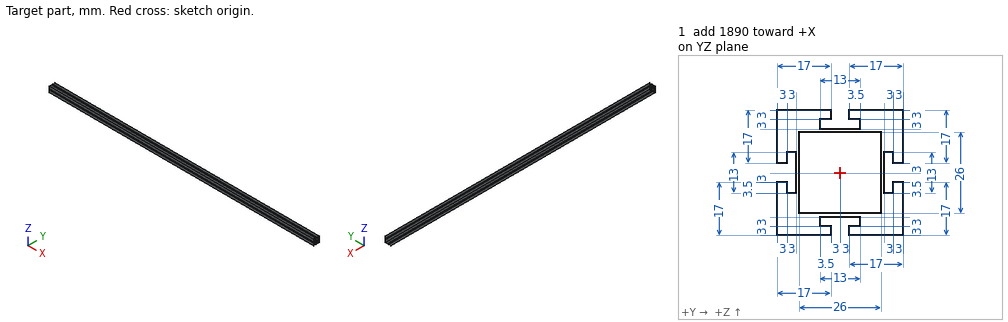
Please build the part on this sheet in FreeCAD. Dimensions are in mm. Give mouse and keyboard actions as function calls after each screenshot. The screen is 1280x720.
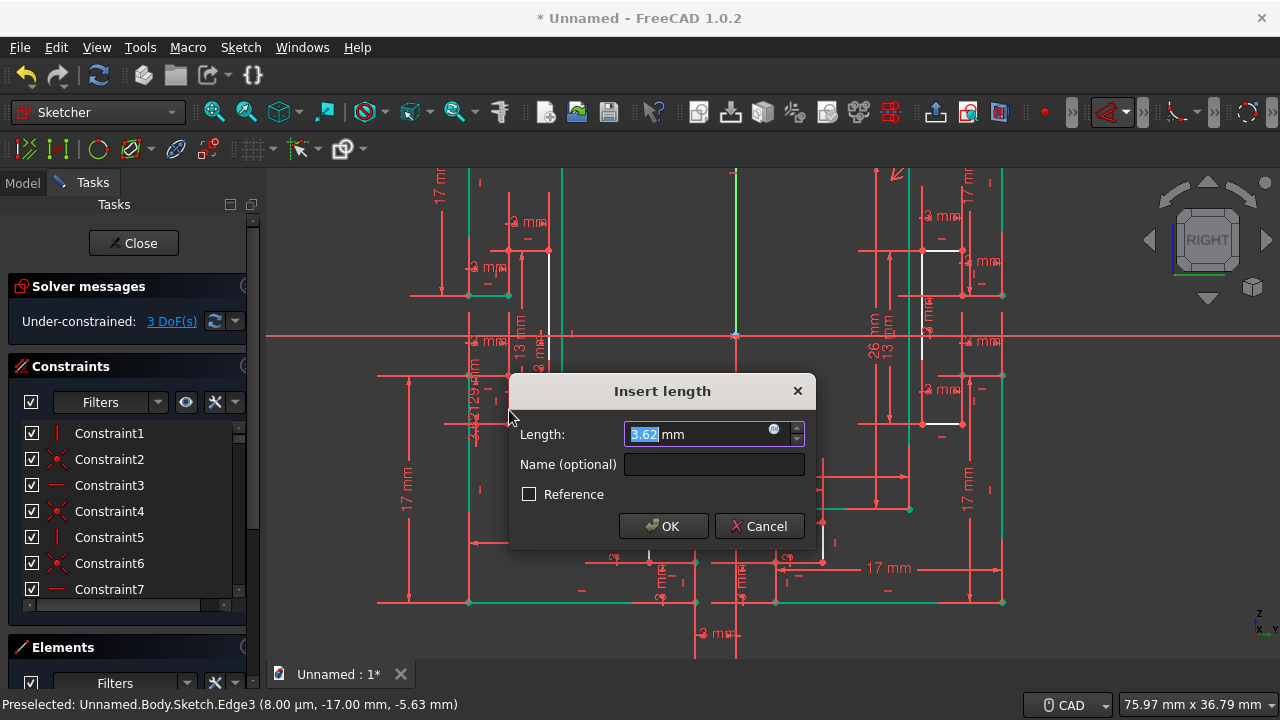
text(3.5)
key(Return)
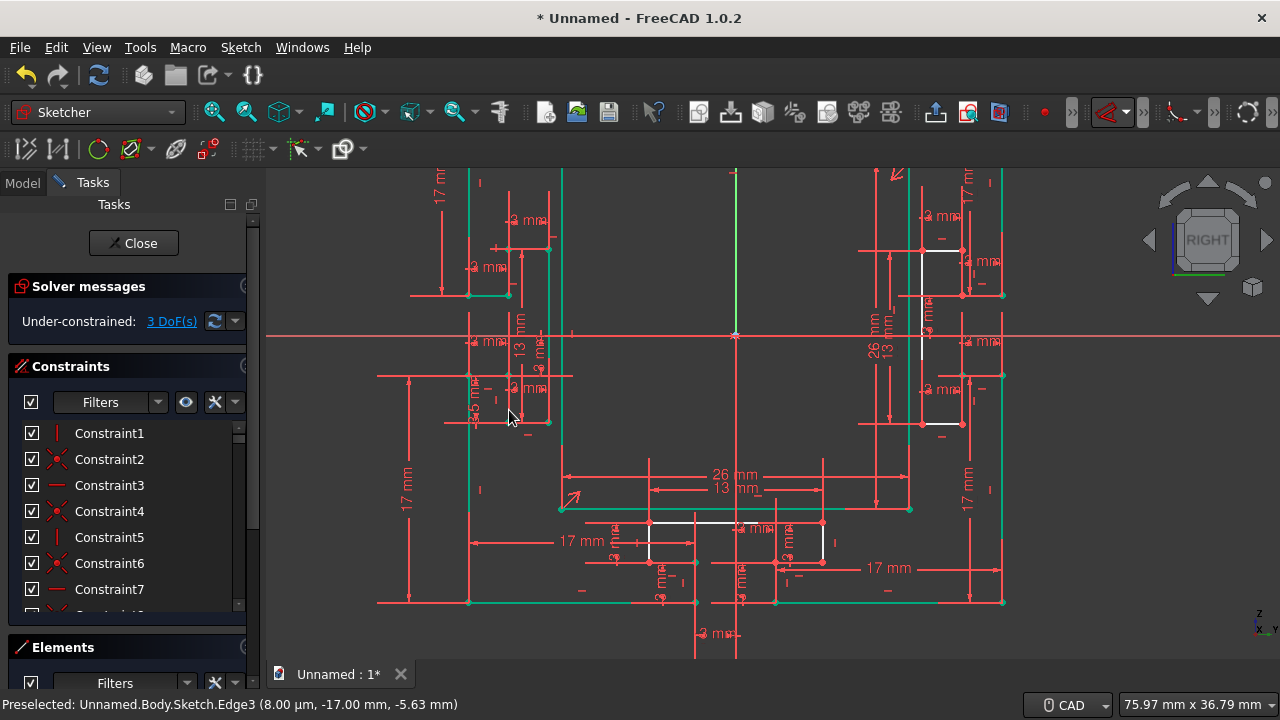
click(682, 563)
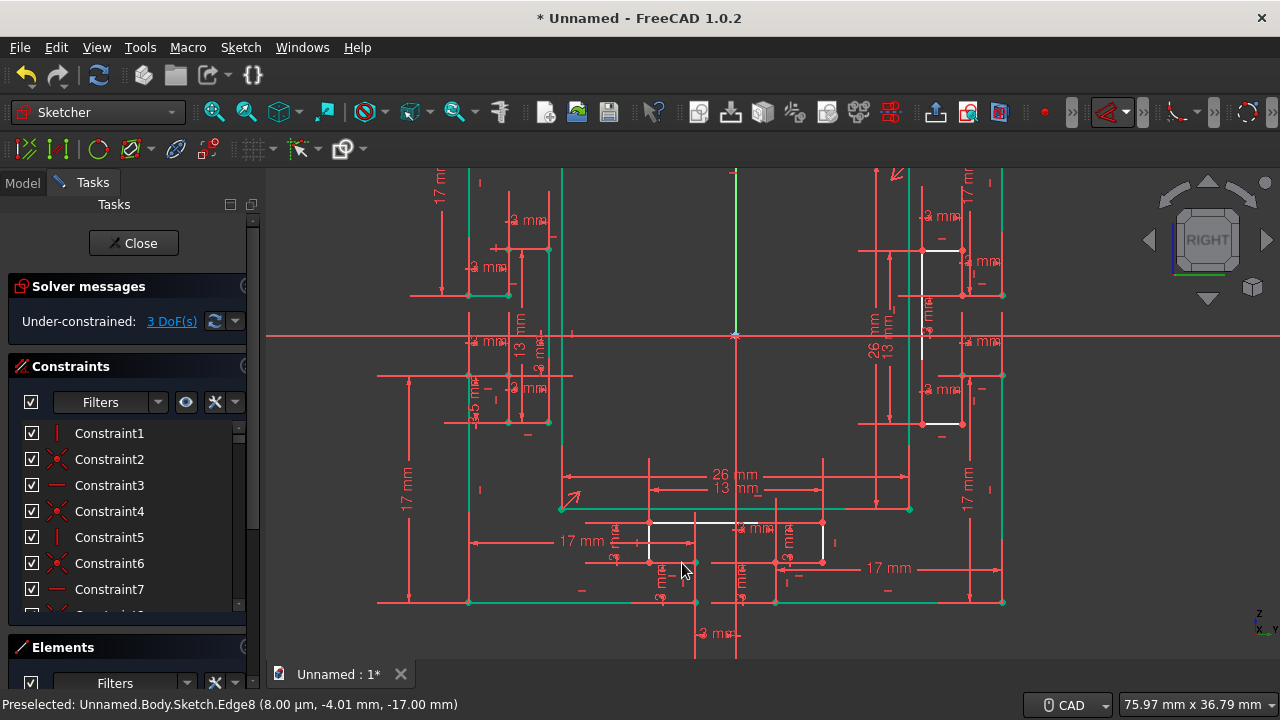
key(l)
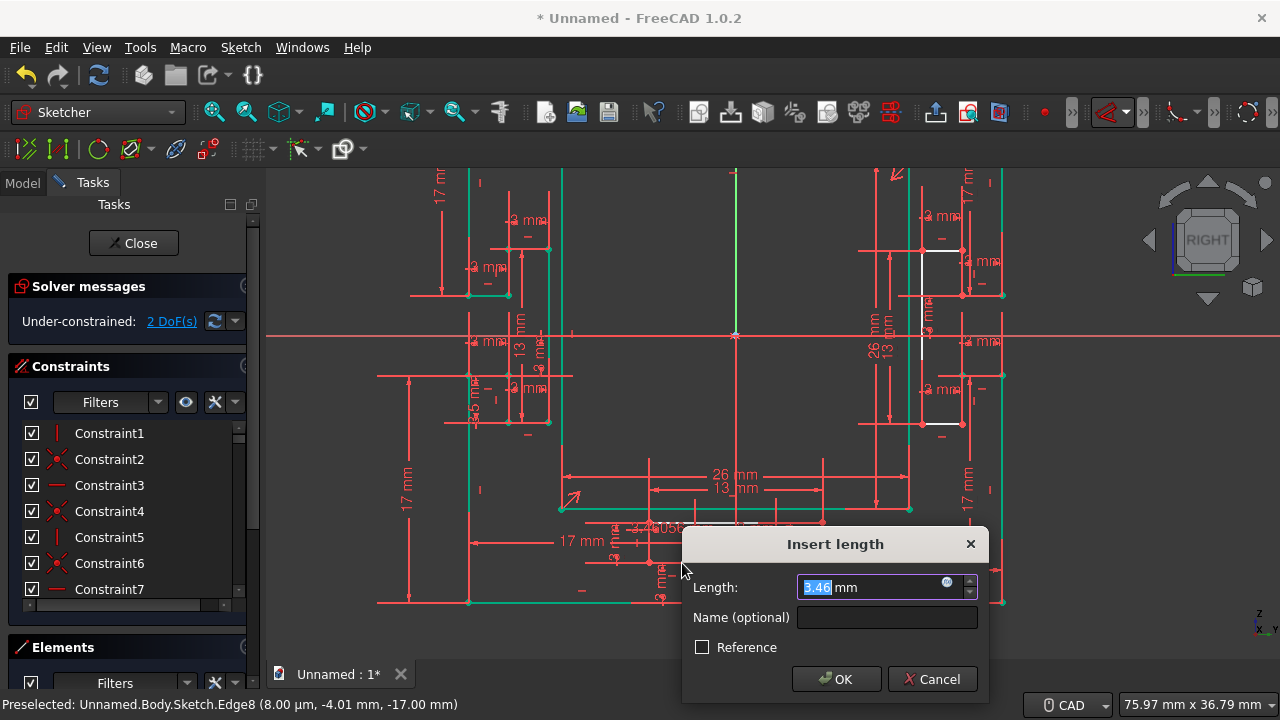
text(3.5)
key(Return)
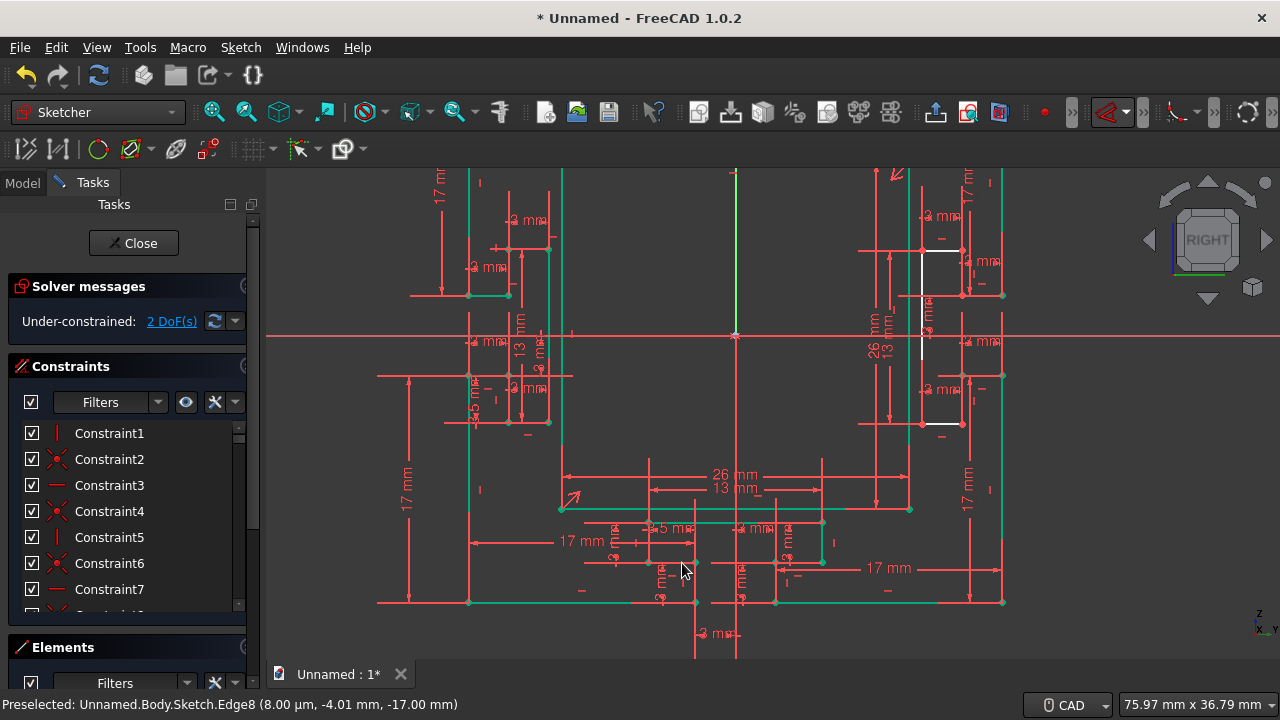
click(962, 390)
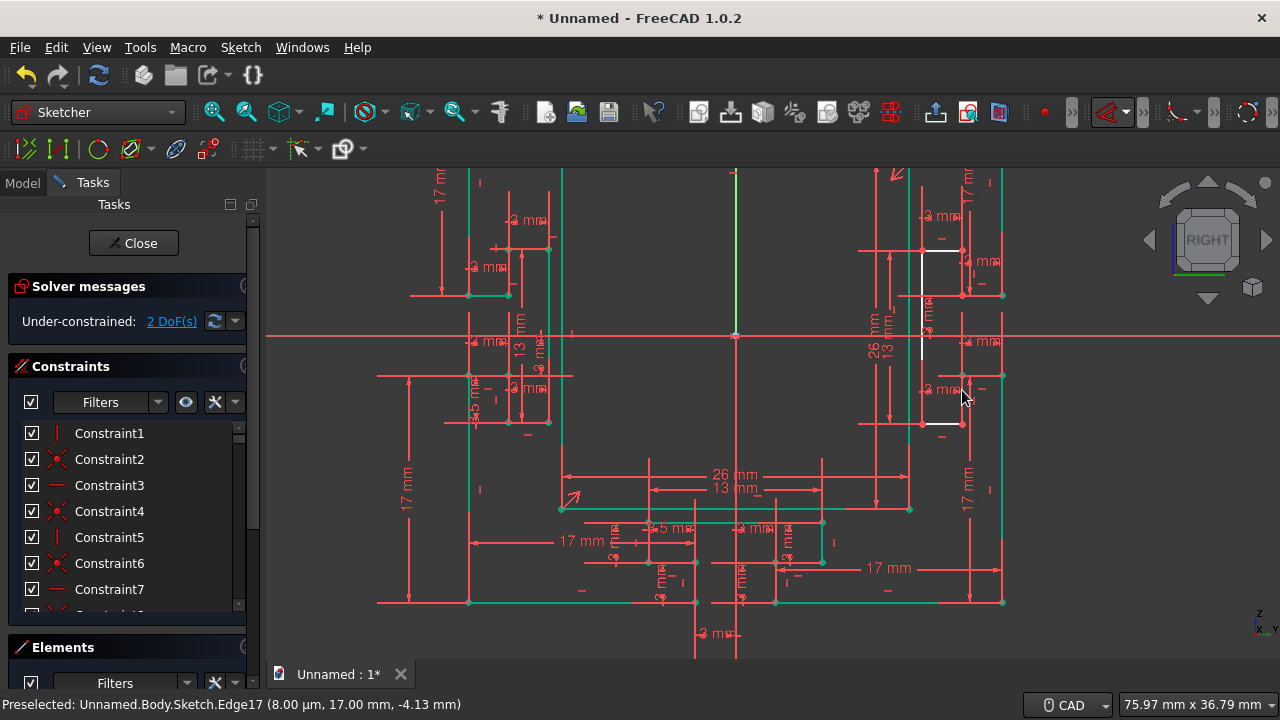
key(i)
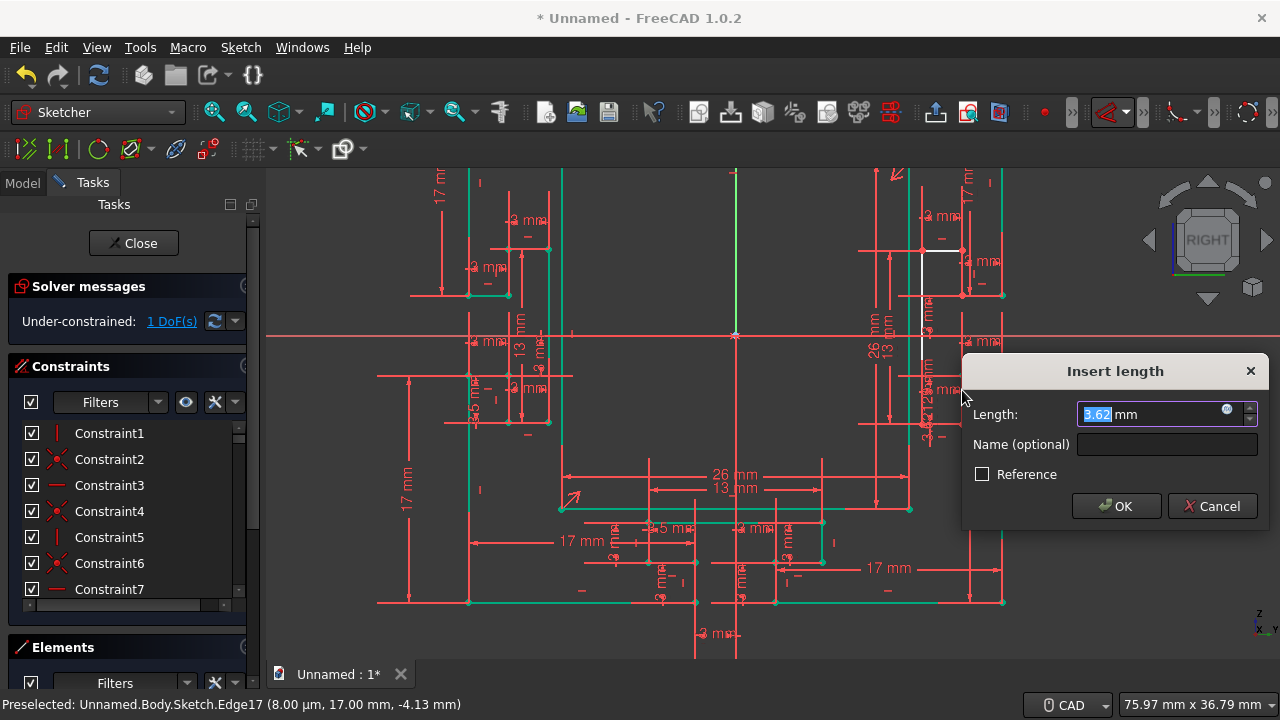
text(3.5)
key(Return)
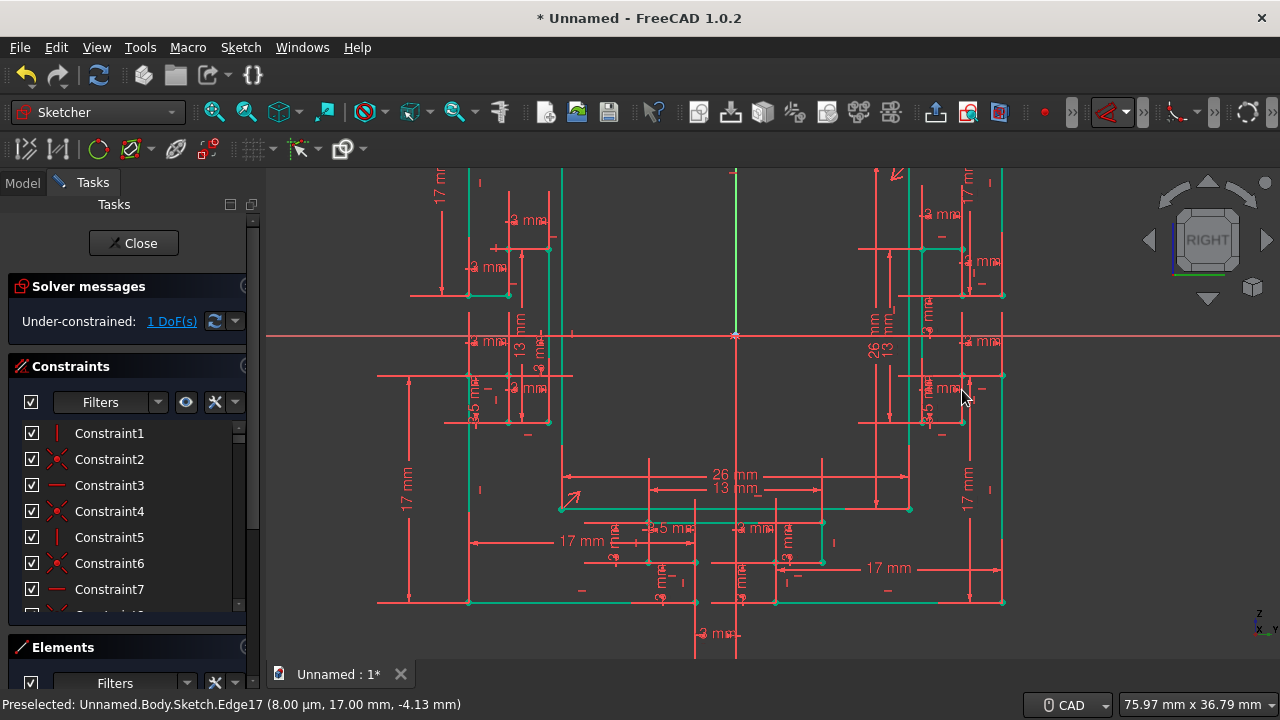
scroll(667, 508, down, 3)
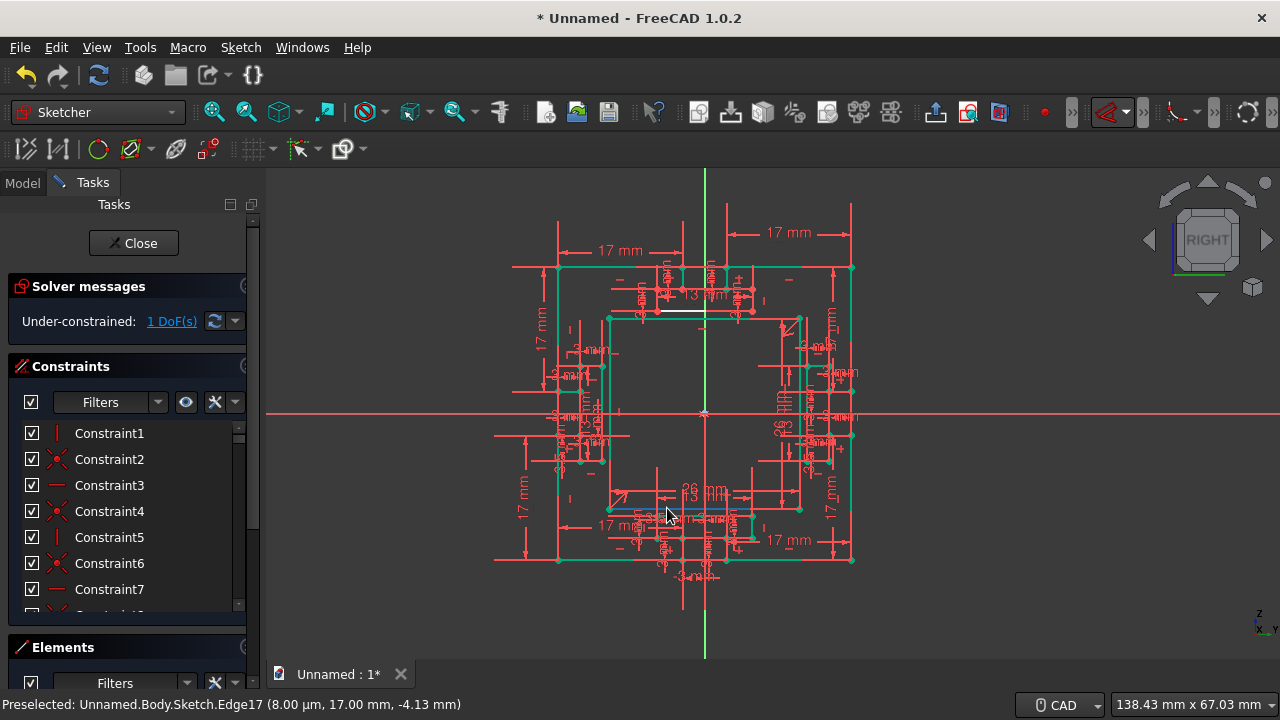
scroll(735, 289, up, 3)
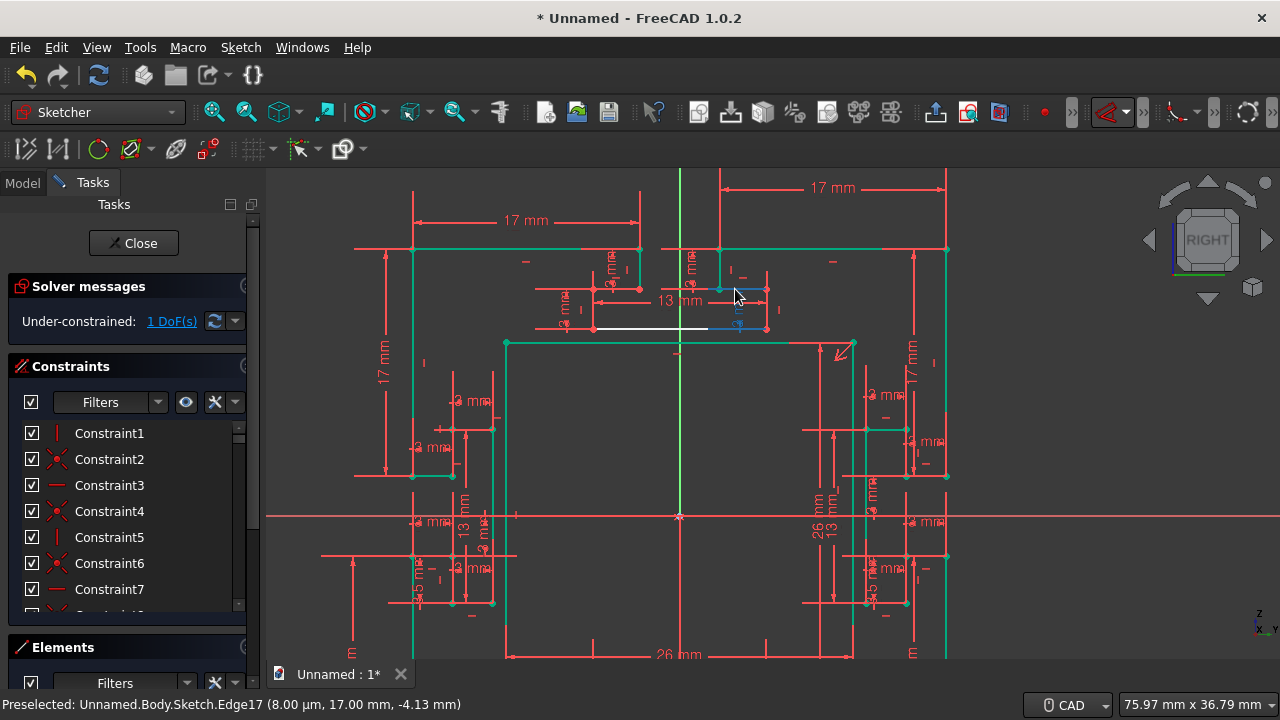
click(734, 289)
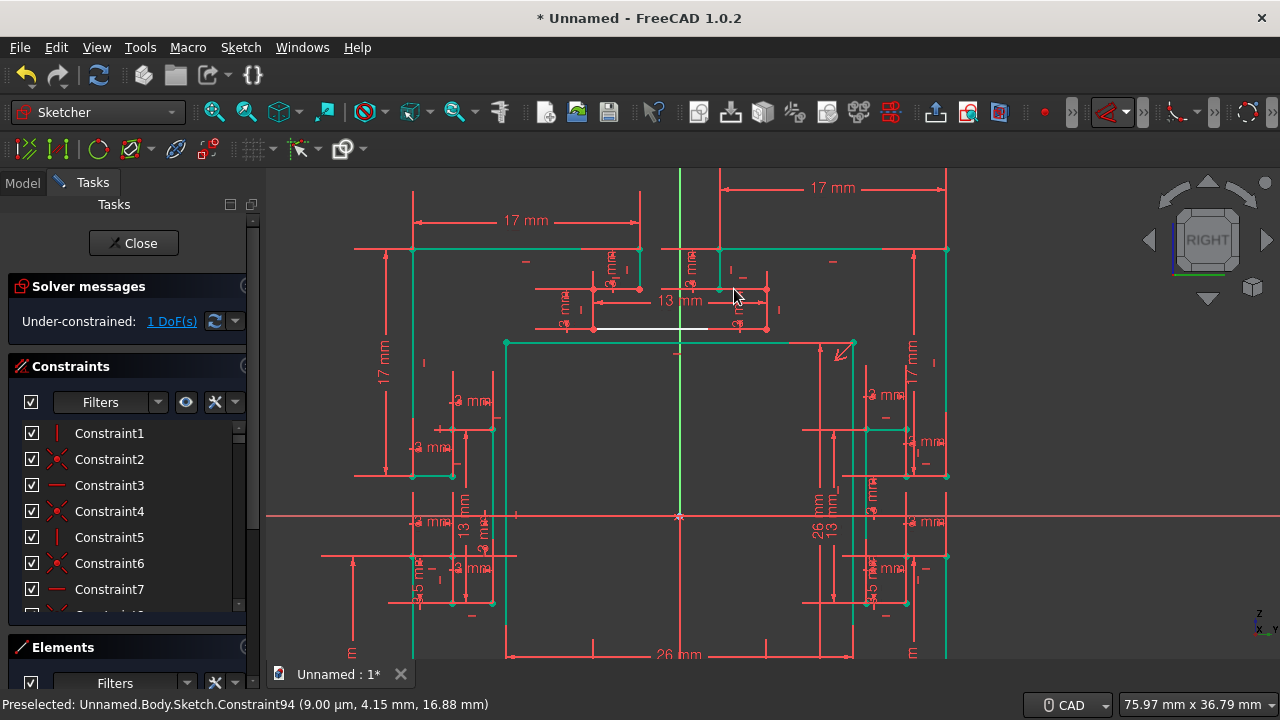
key(l)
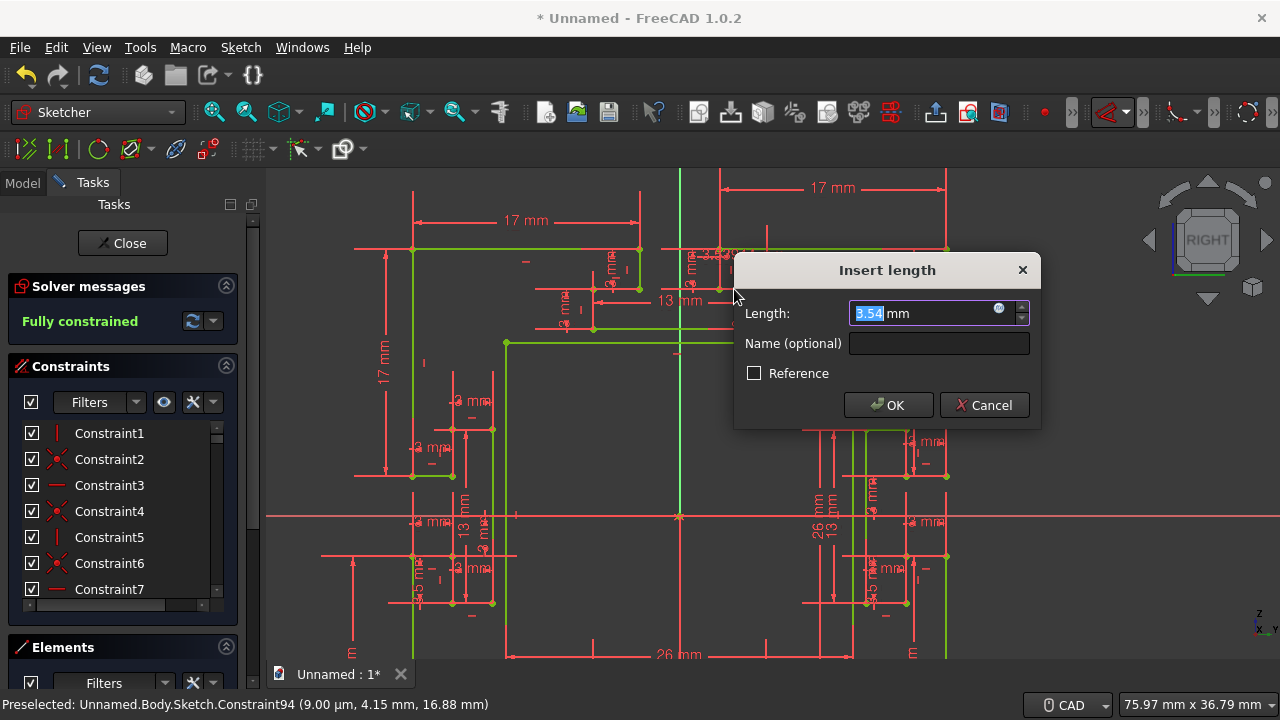
text(3.5)
key(Return)